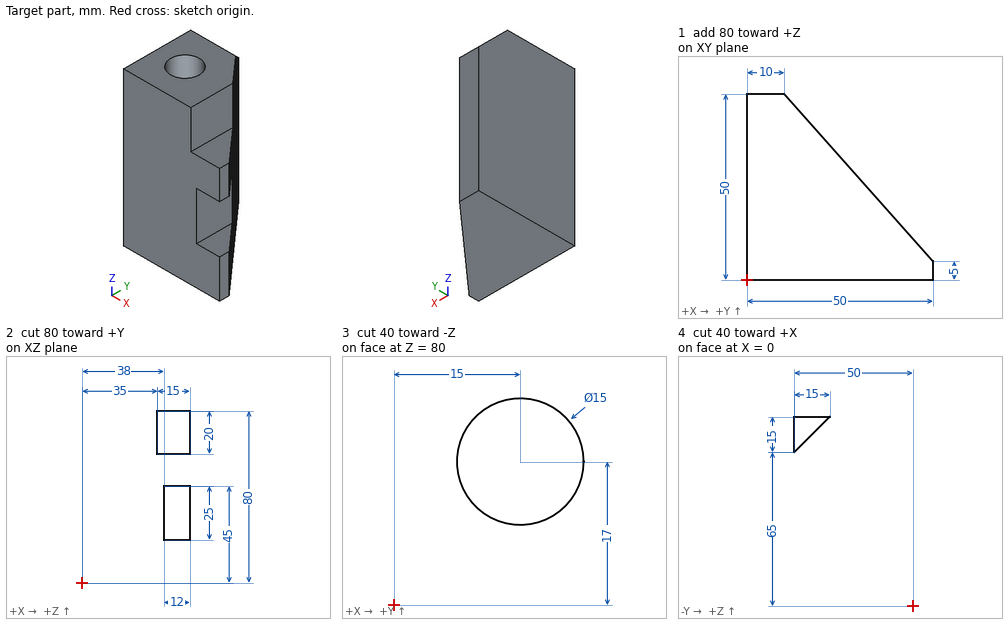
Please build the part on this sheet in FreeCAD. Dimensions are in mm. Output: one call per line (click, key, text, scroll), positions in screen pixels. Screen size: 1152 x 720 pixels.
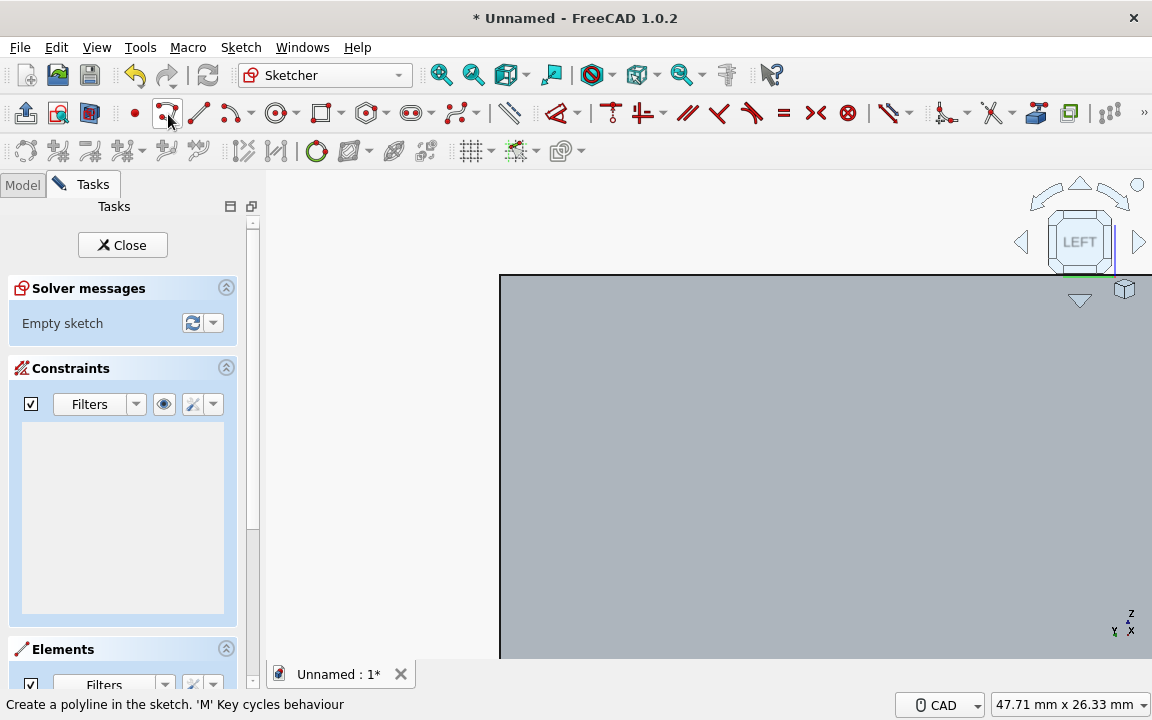
click(500, 553)
click(779, 275)
click(500, 275)
click(500, 554)
key(Escape)
key(Escape)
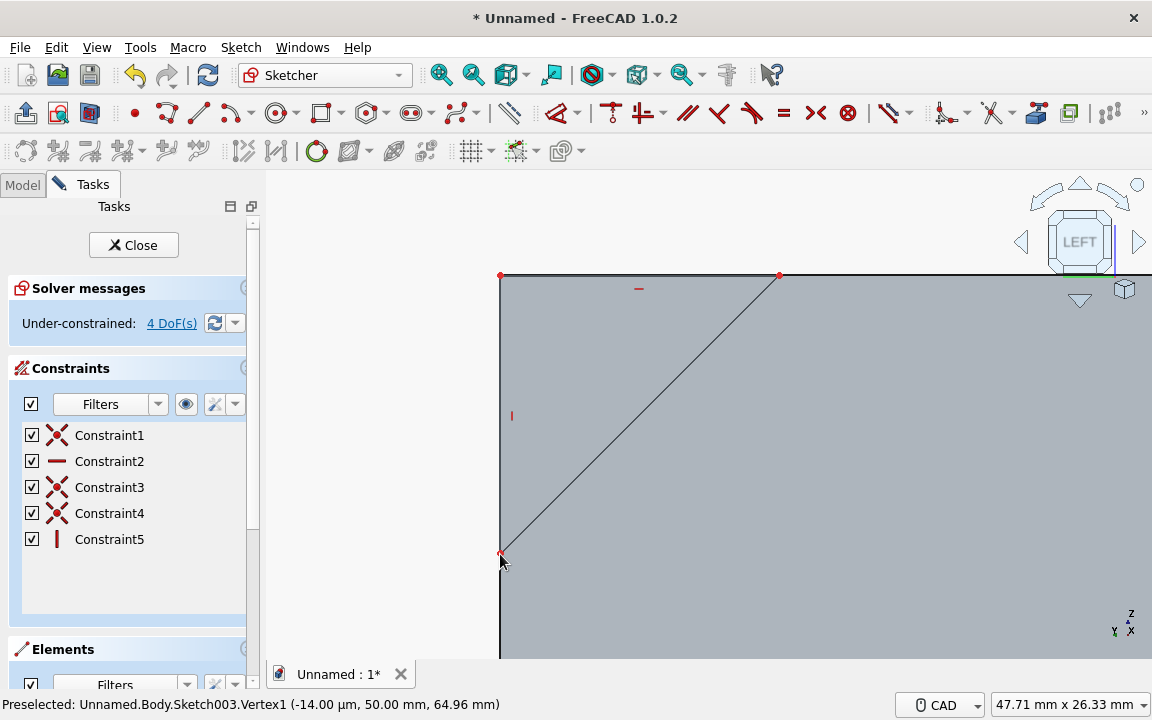
click(556, 114)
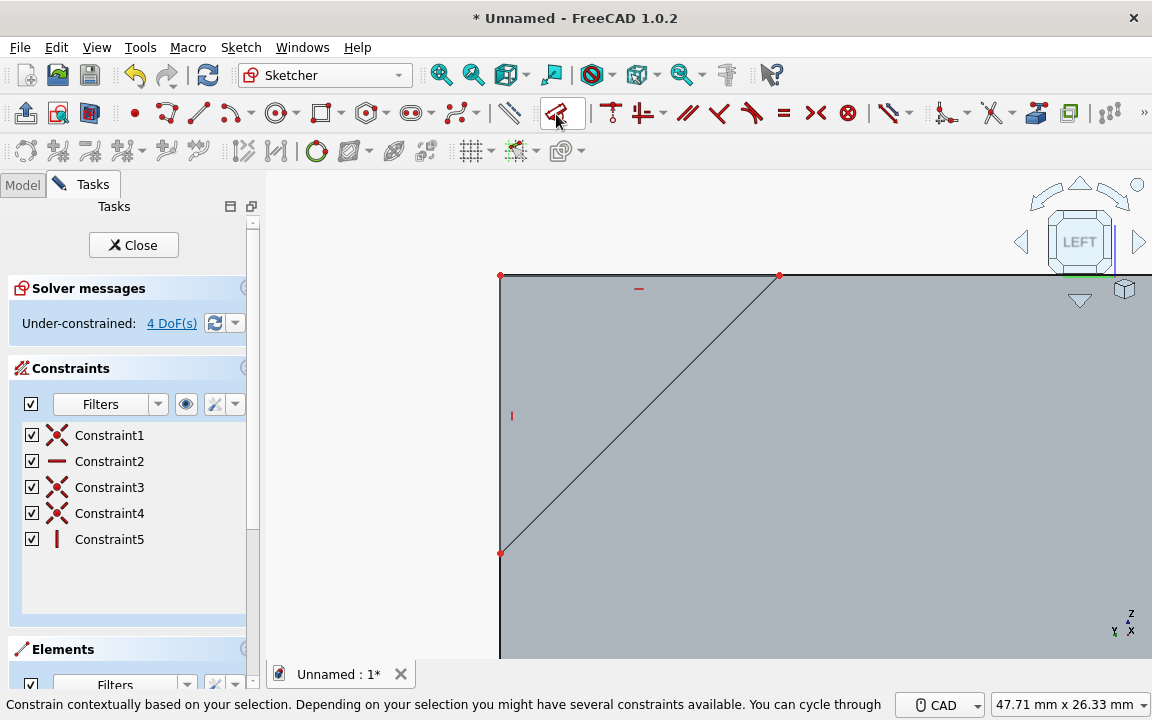
click(695, 276)
click(639, 242)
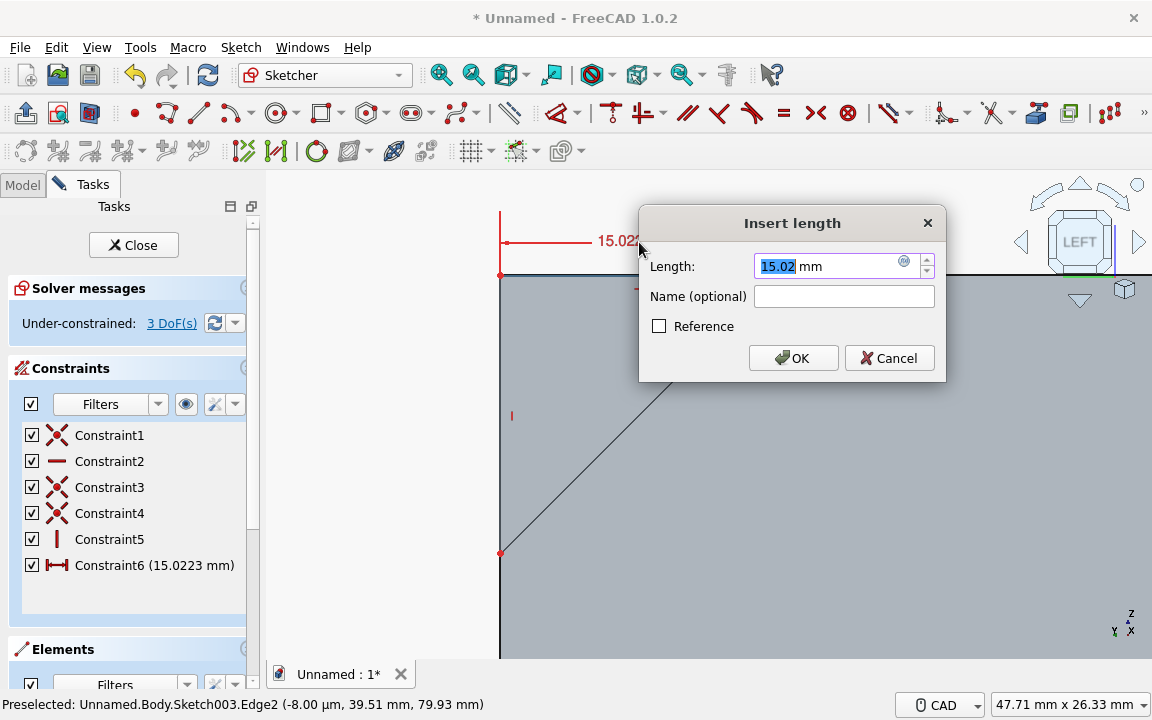
text(15)
key(Return)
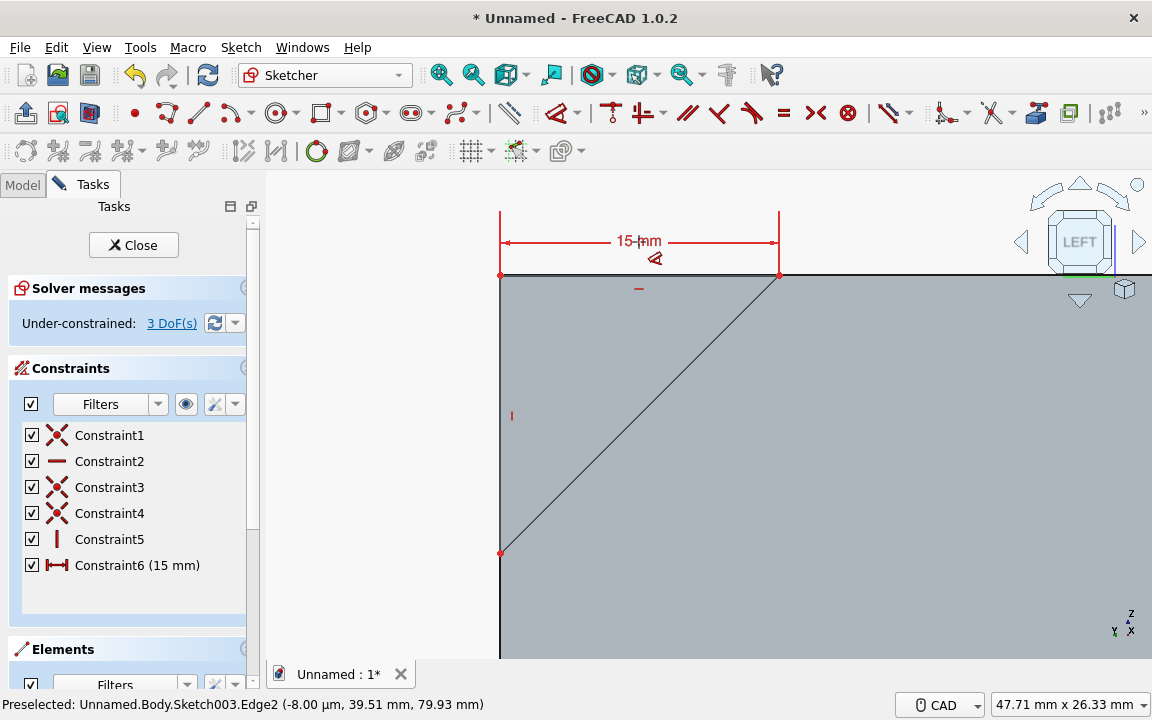
click(500, 359)
click(466, 415)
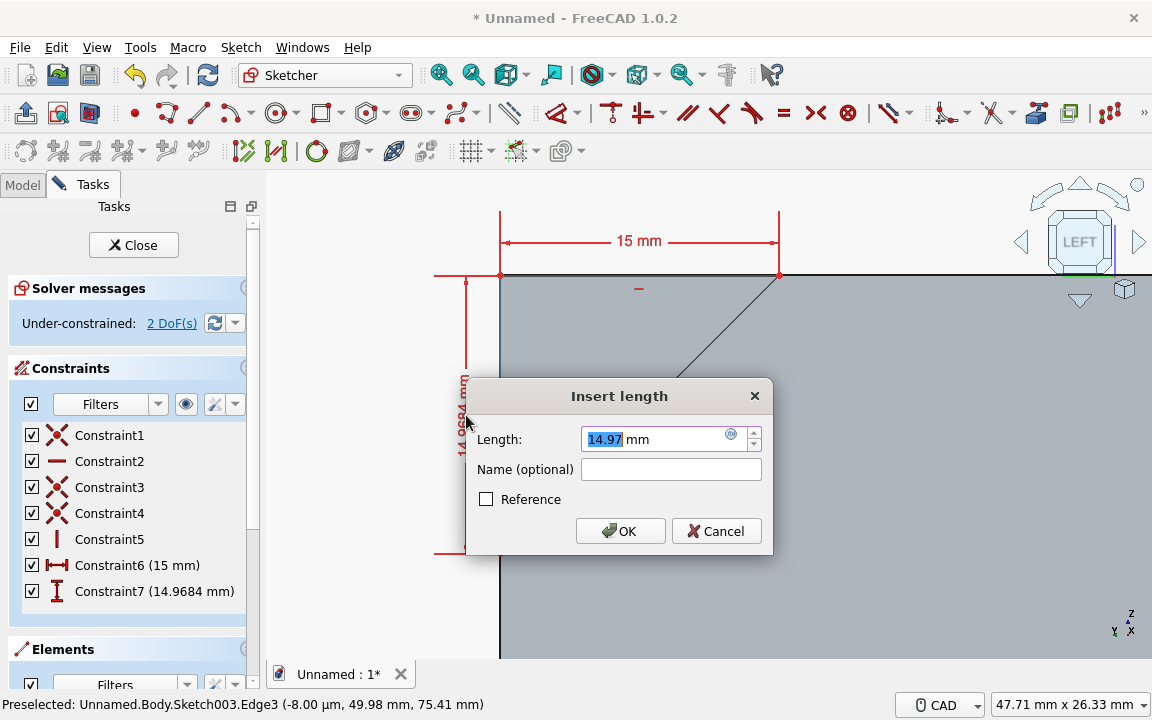
text(15)
key(Return)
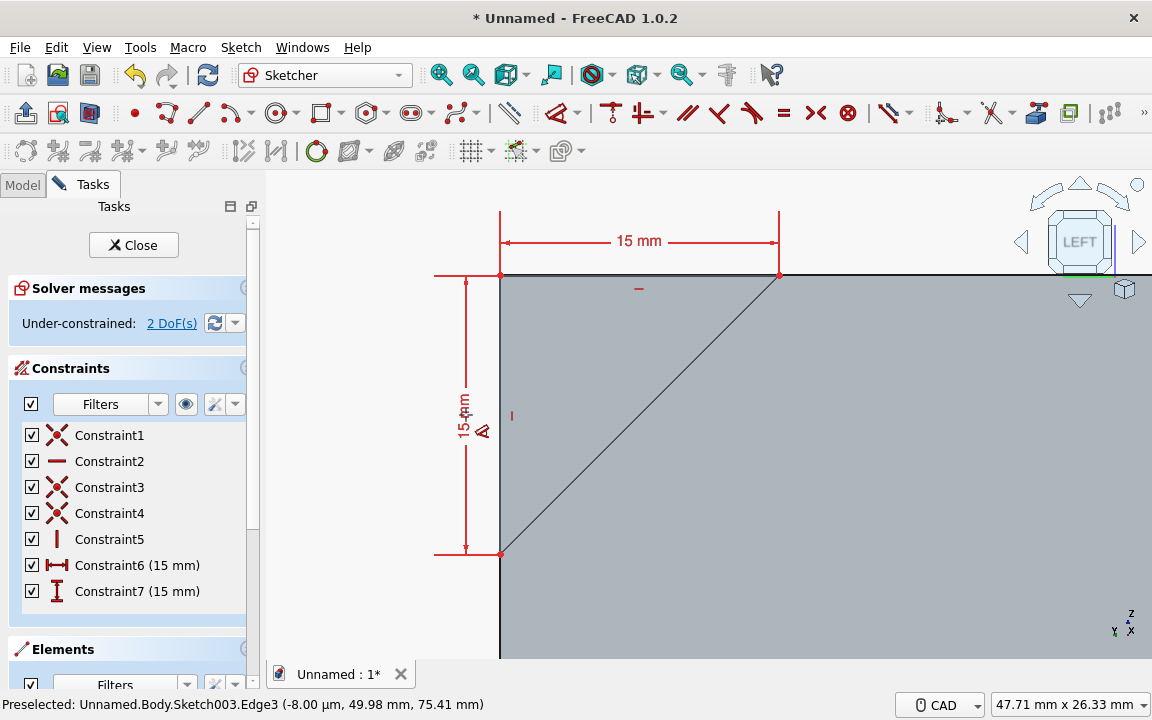
click(500, 555)
click(744, 521)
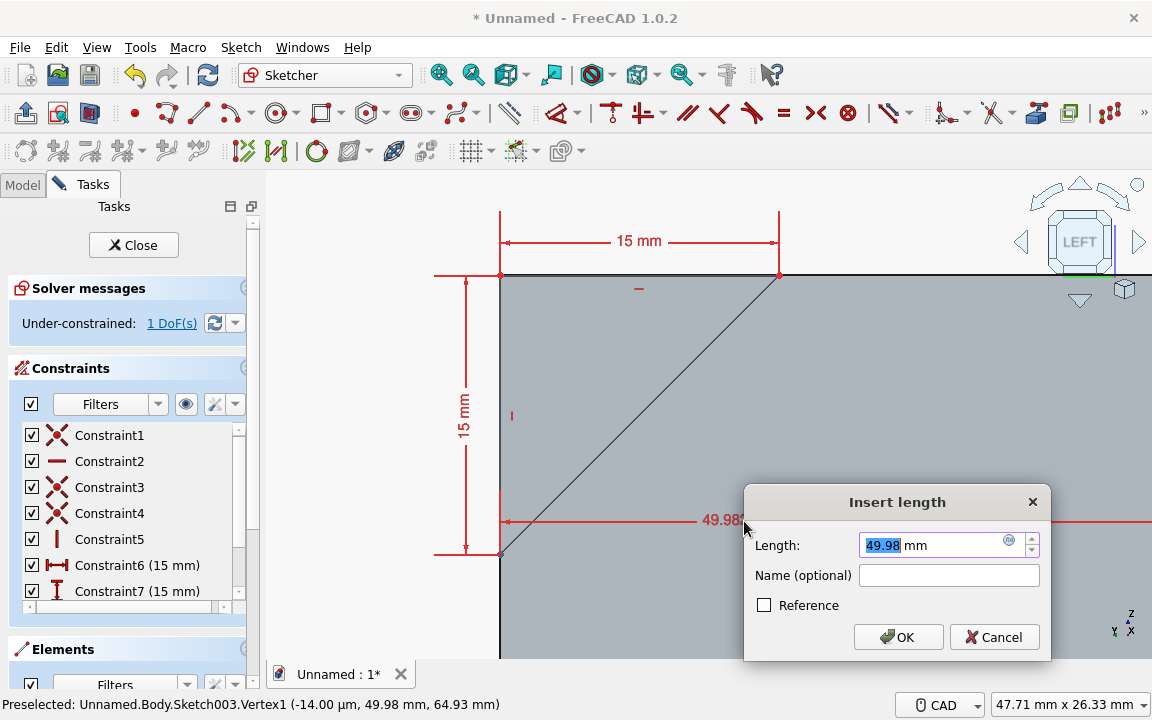
text(50)
key(Return)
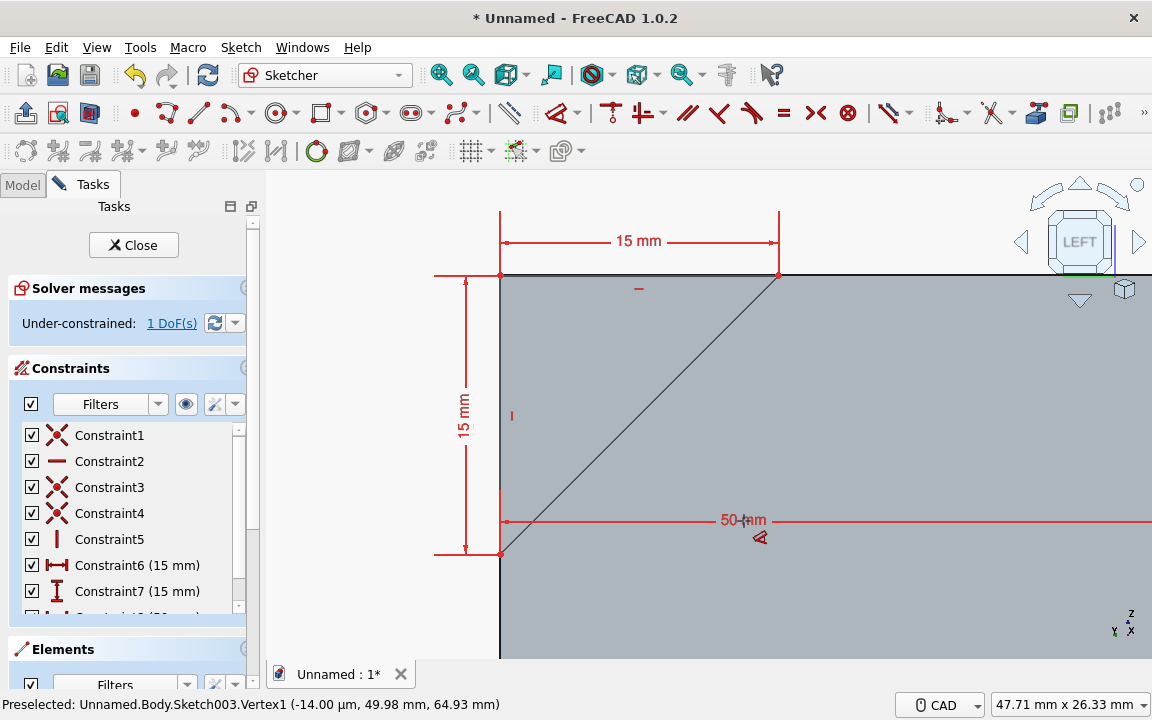
click(500, 555)
click(466, 593)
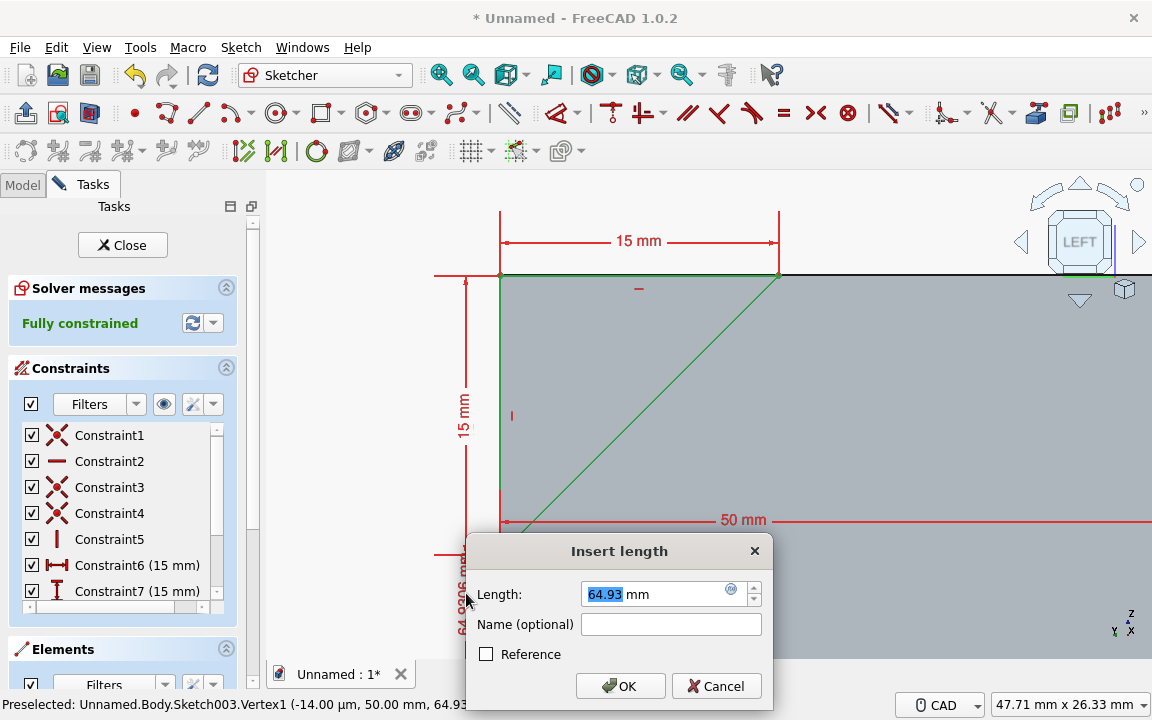
text(65)
key(Return)
key(Escape)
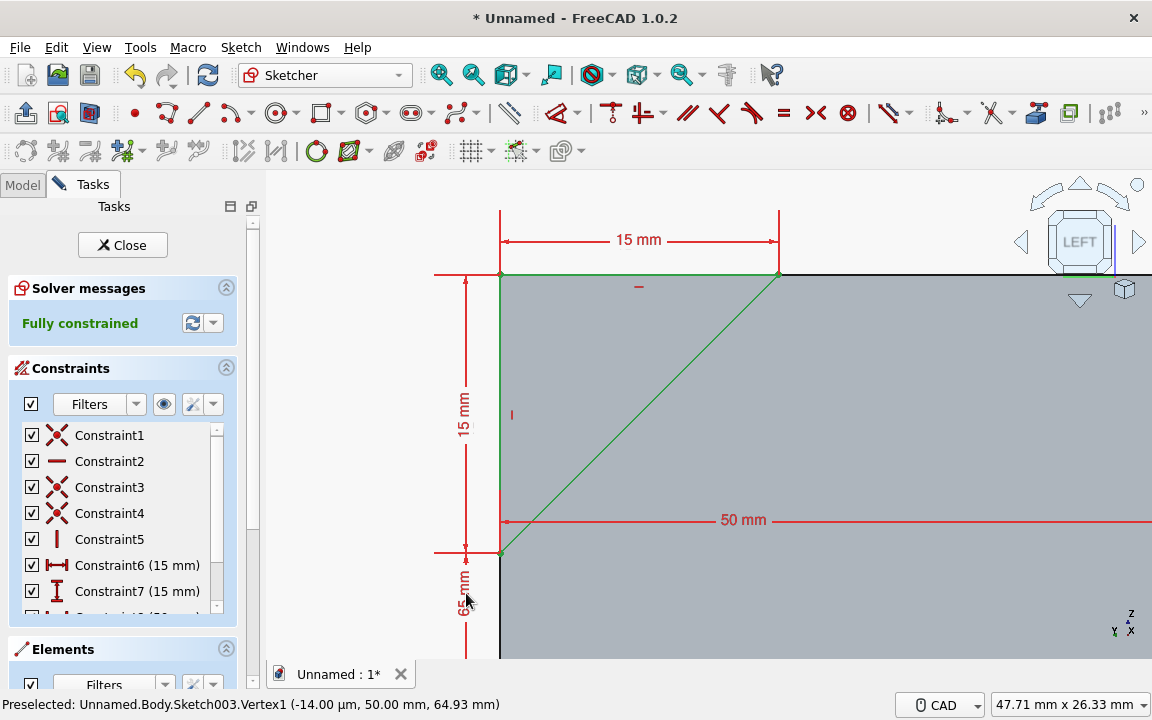
click(123, 245)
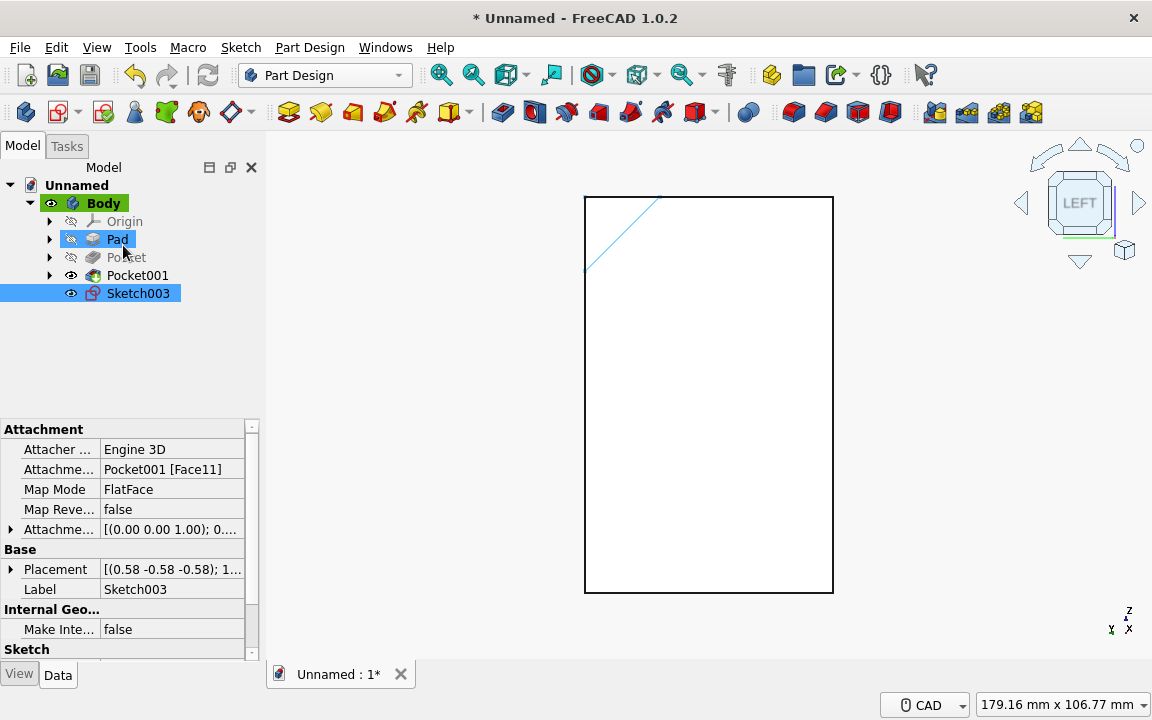
click(504, 112)